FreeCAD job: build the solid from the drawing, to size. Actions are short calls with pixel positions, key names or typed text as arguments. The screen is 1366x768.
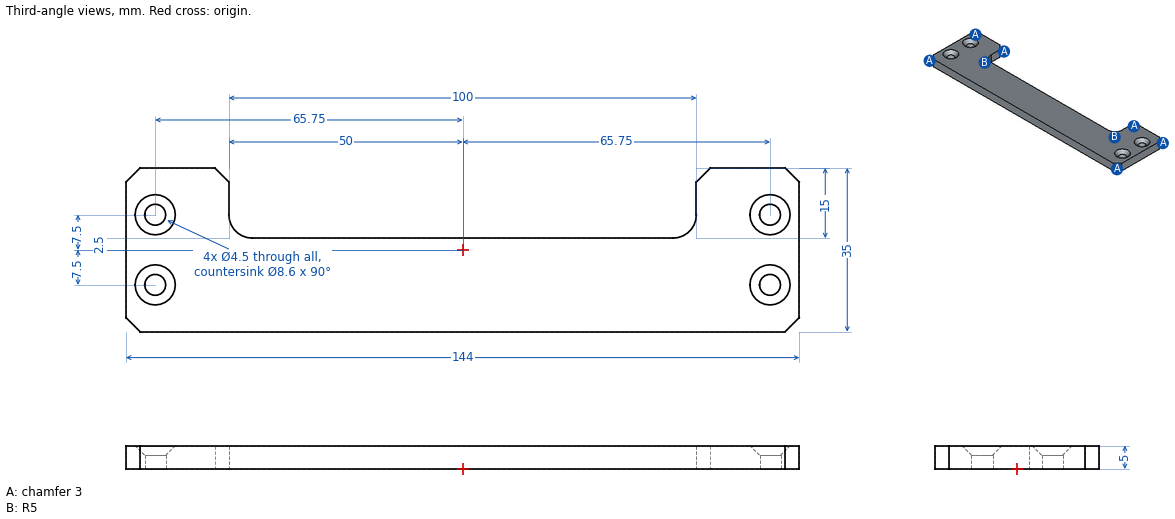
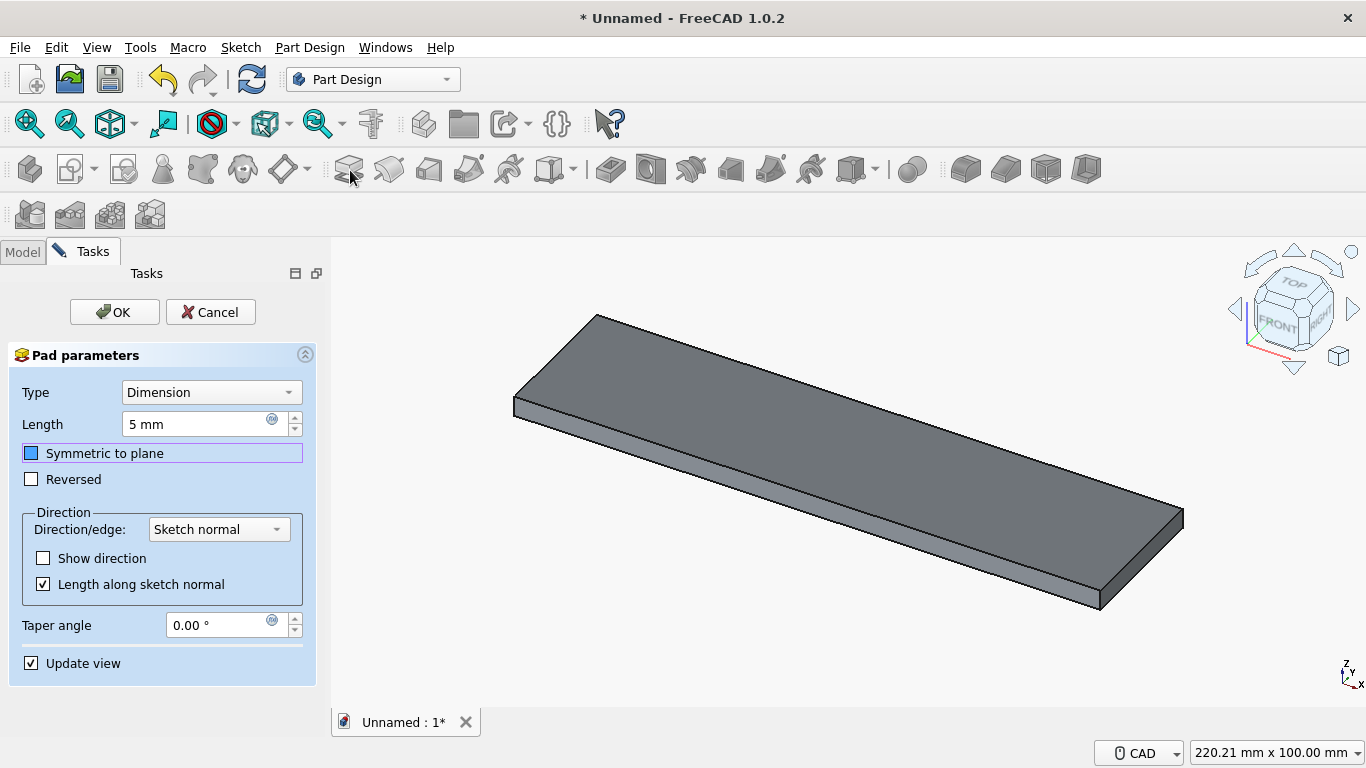
click(115, 312)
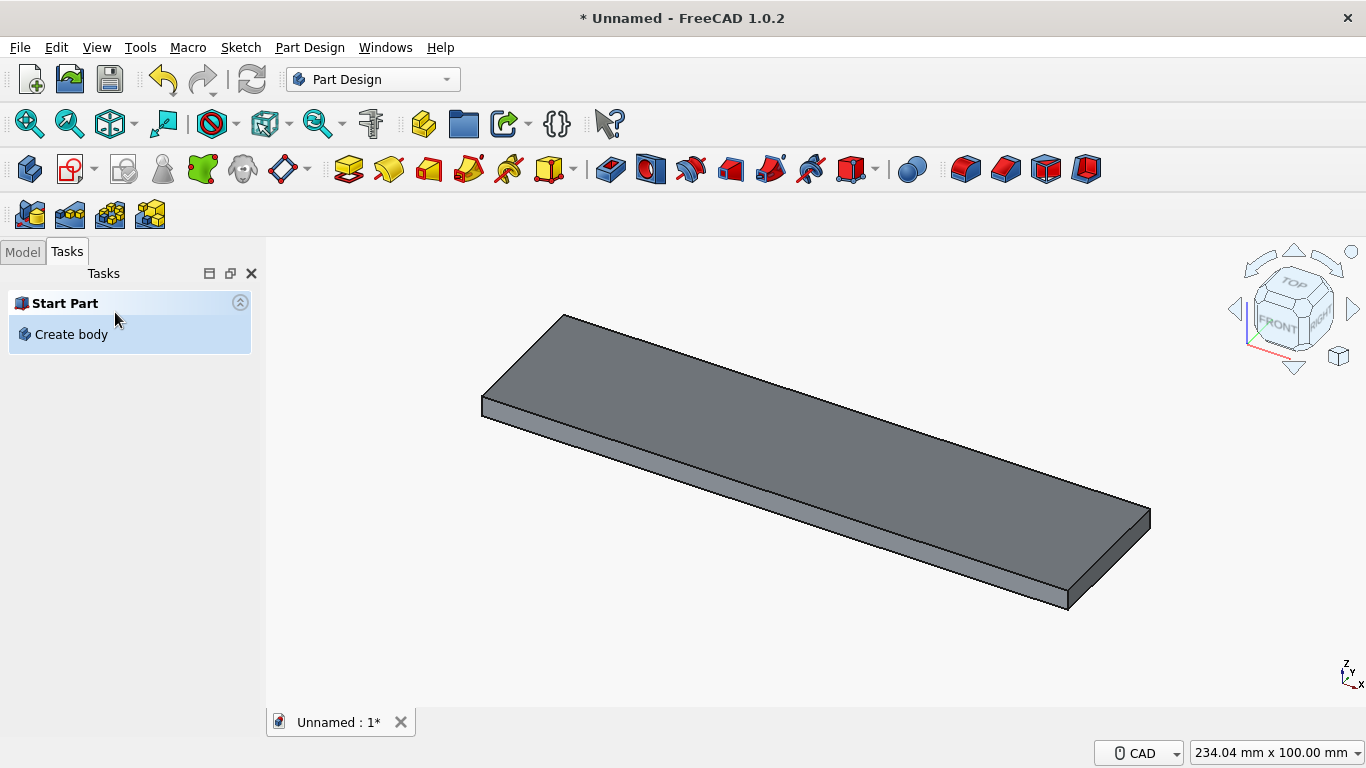
click(983, 507)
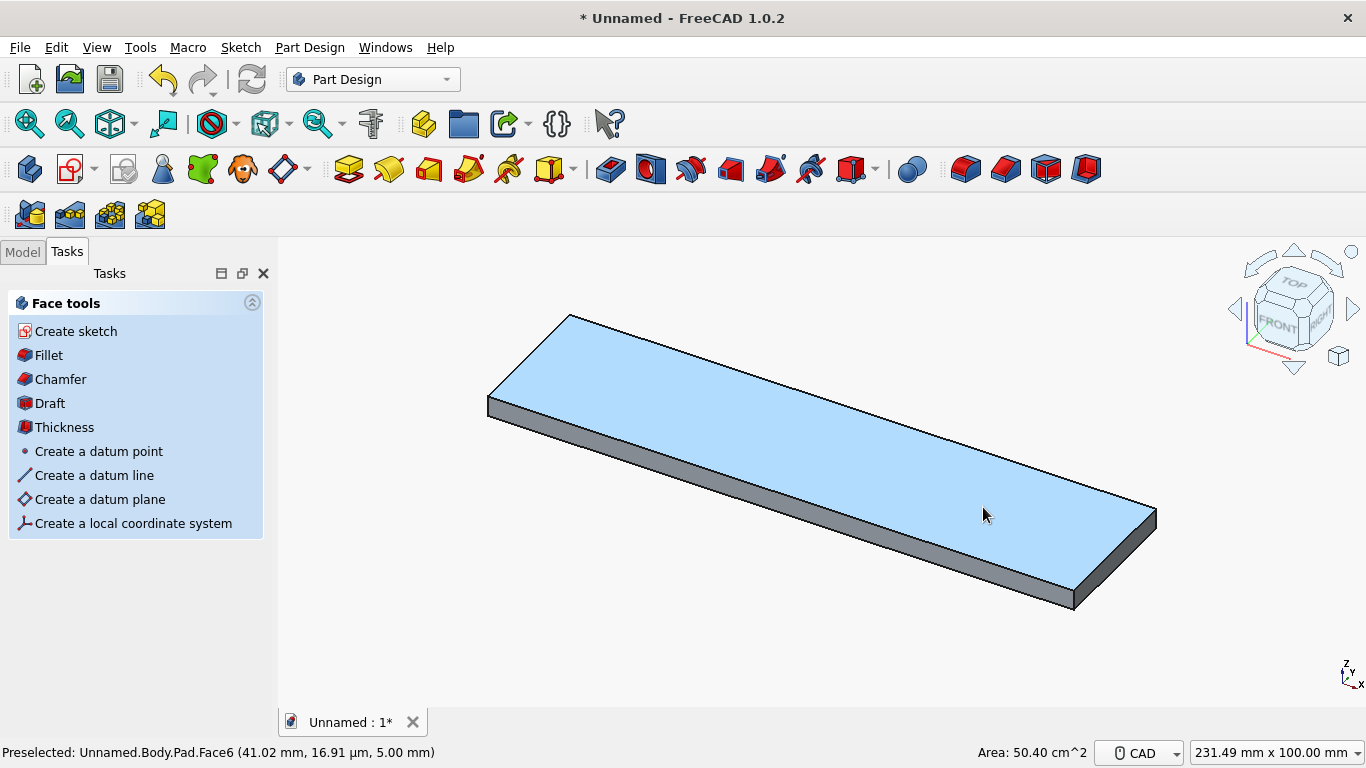
click(70, 170)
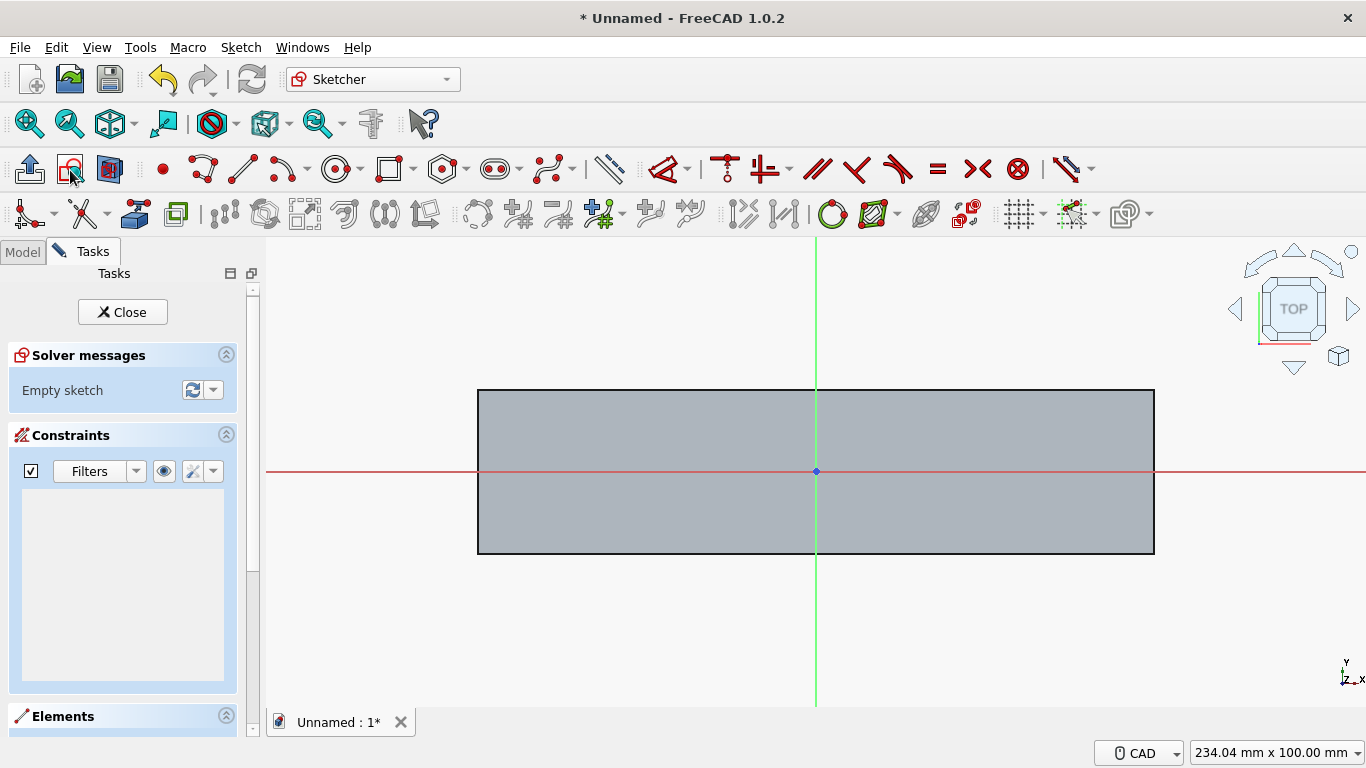
key(g)
key(c)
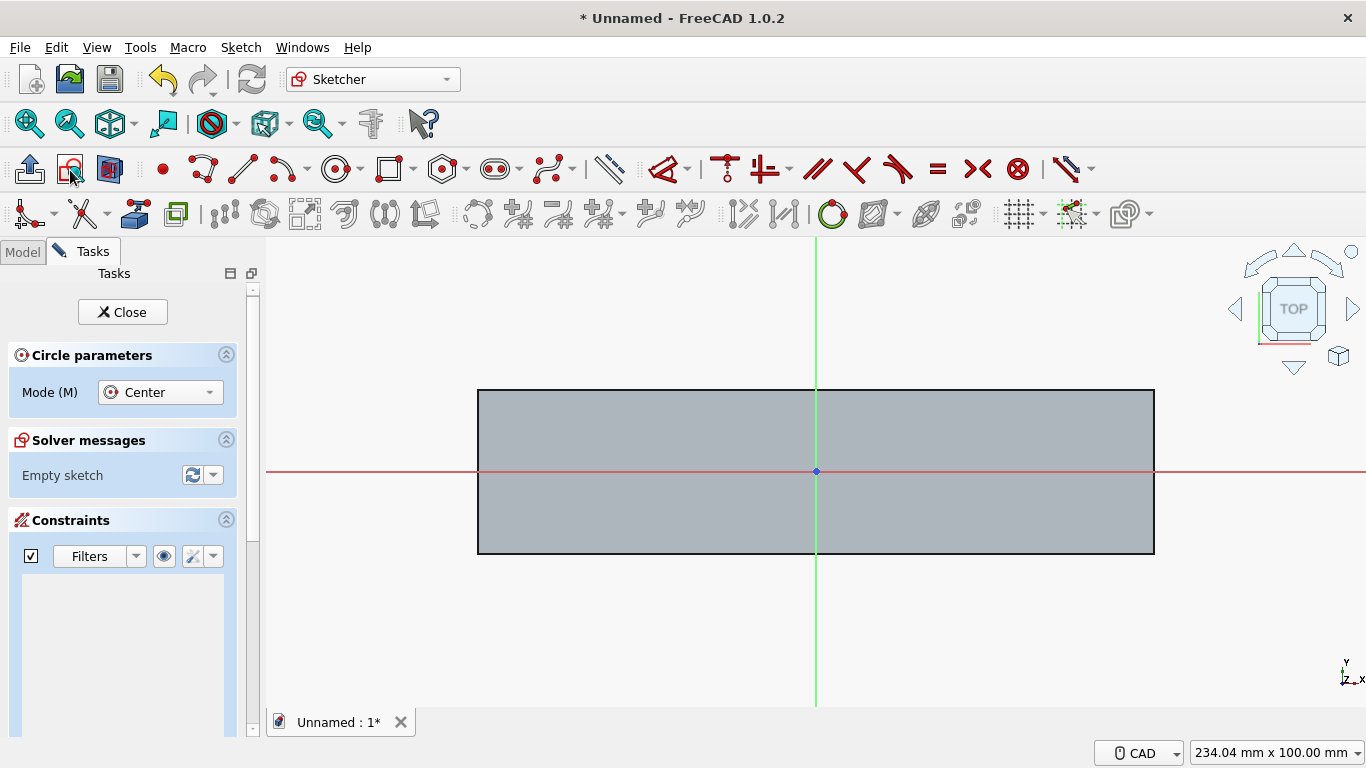
scroll(507, 437, up, 4)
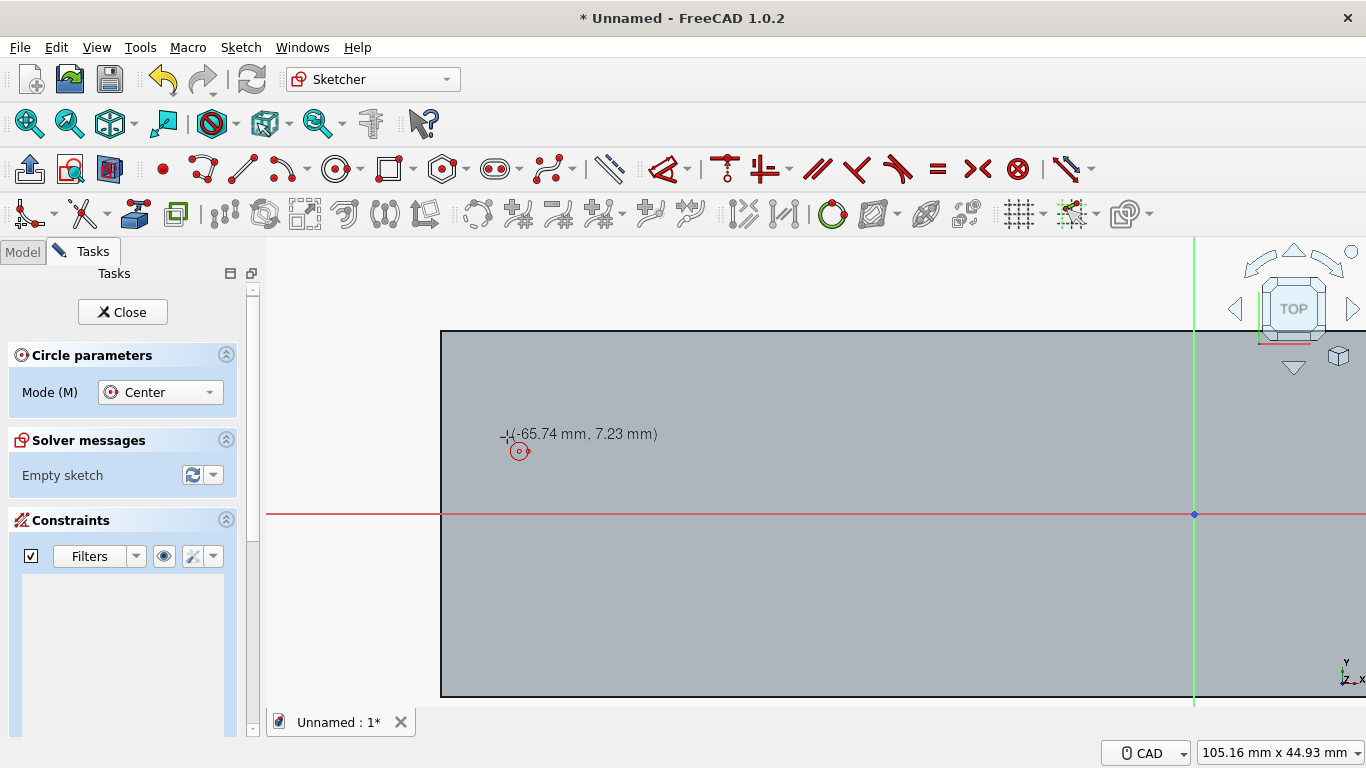
click(507, 436)
move(523, 419)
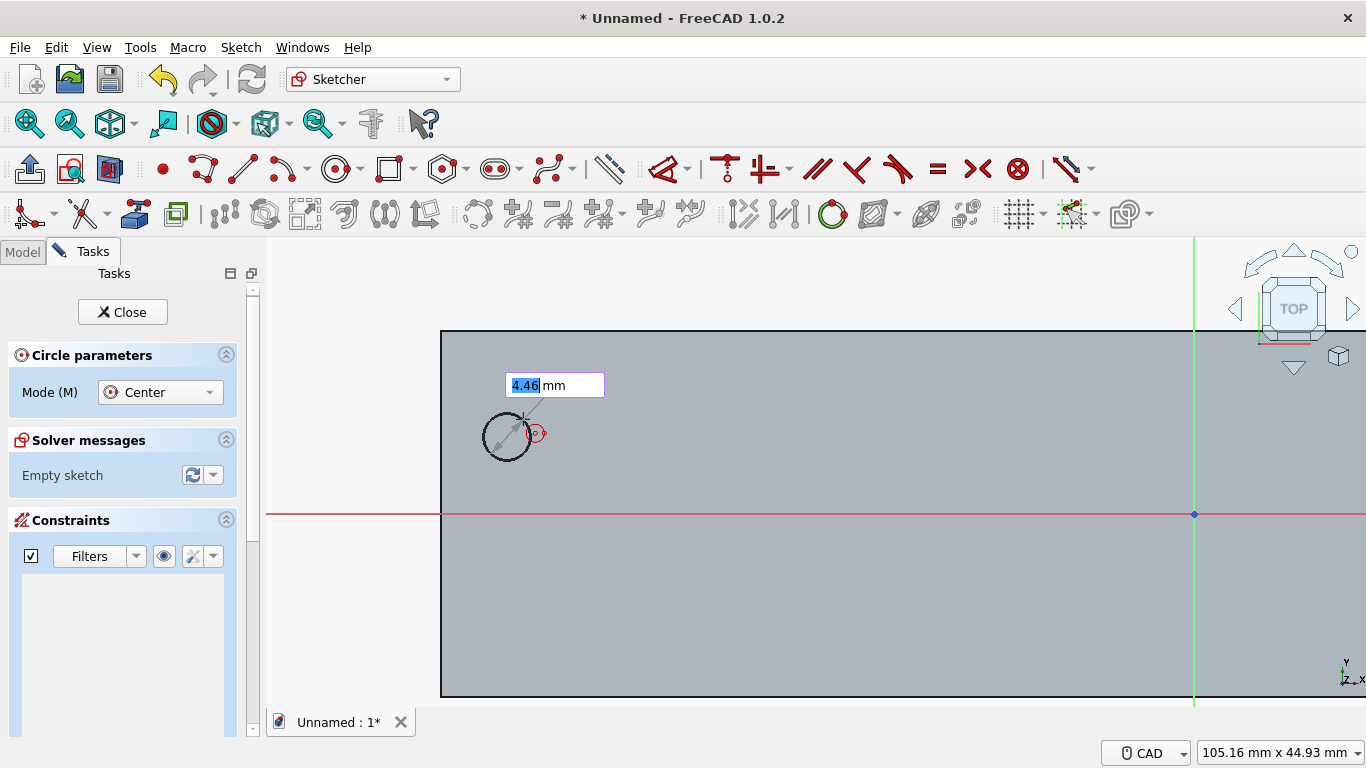
text(4.5)
key(Return)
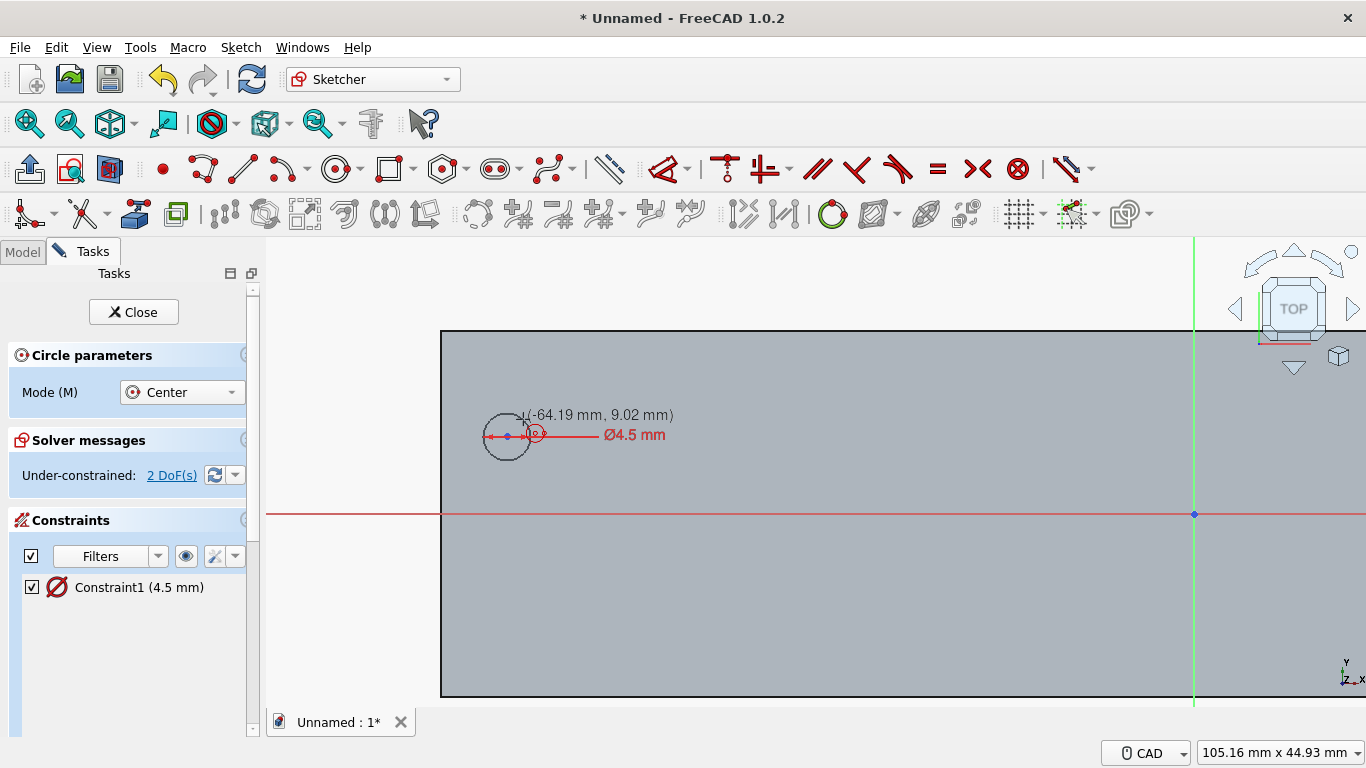
click(507, 593)
move(523, 576)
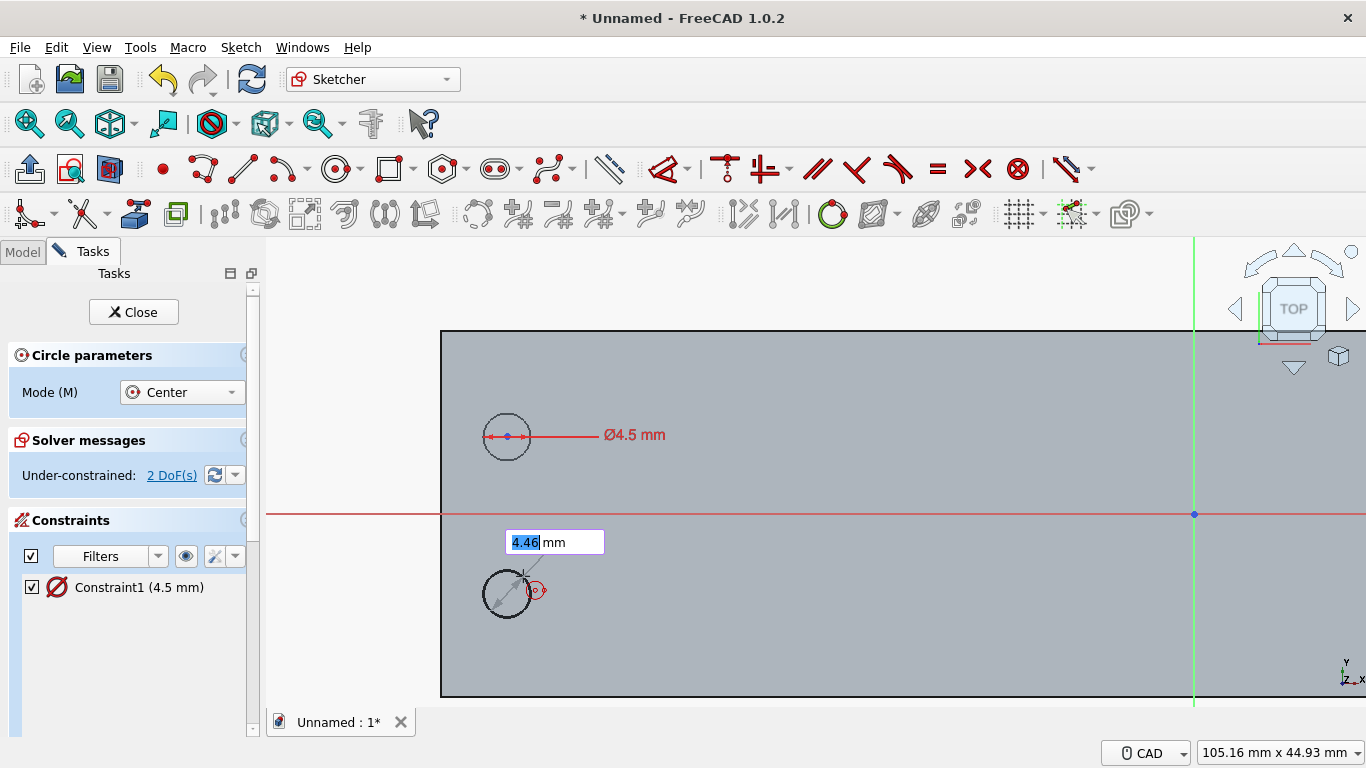
text(4.5)
key(Return)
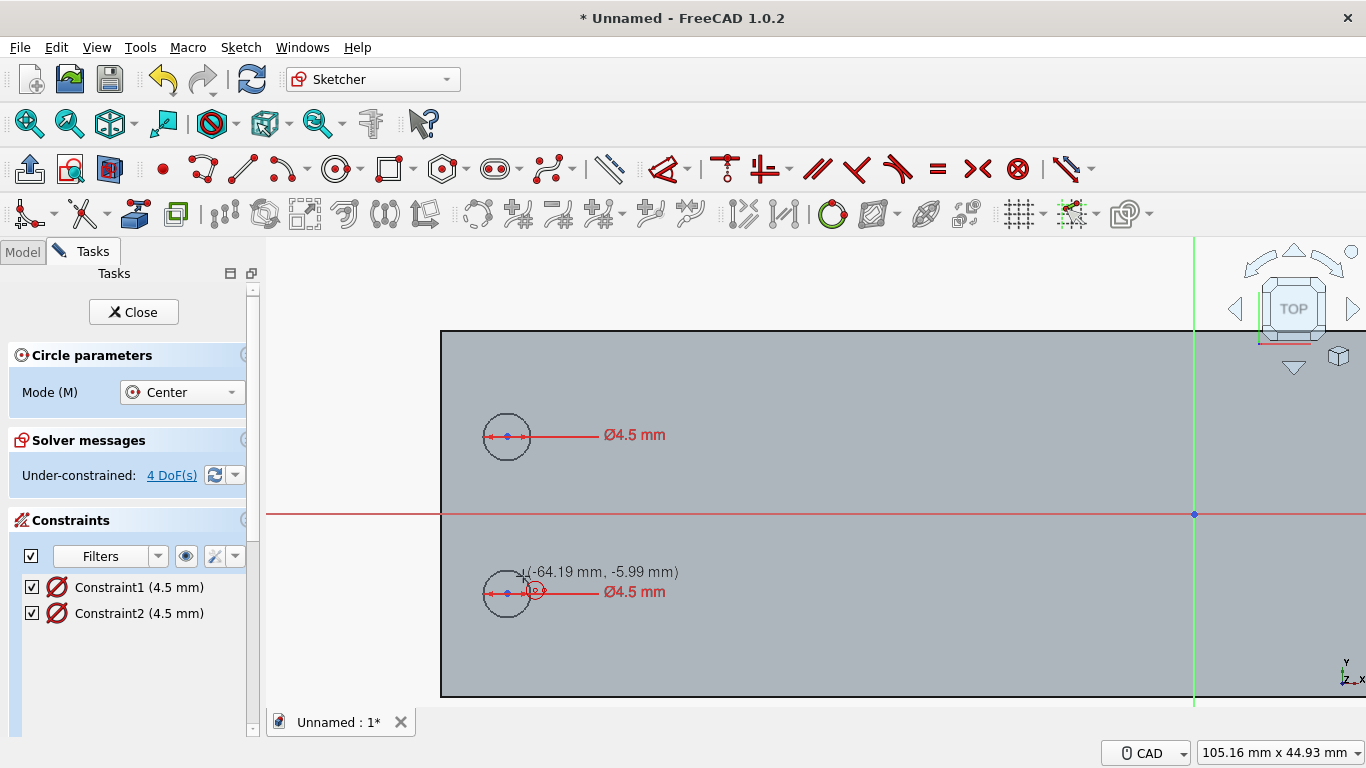
scroll(383, 437, down, 4)